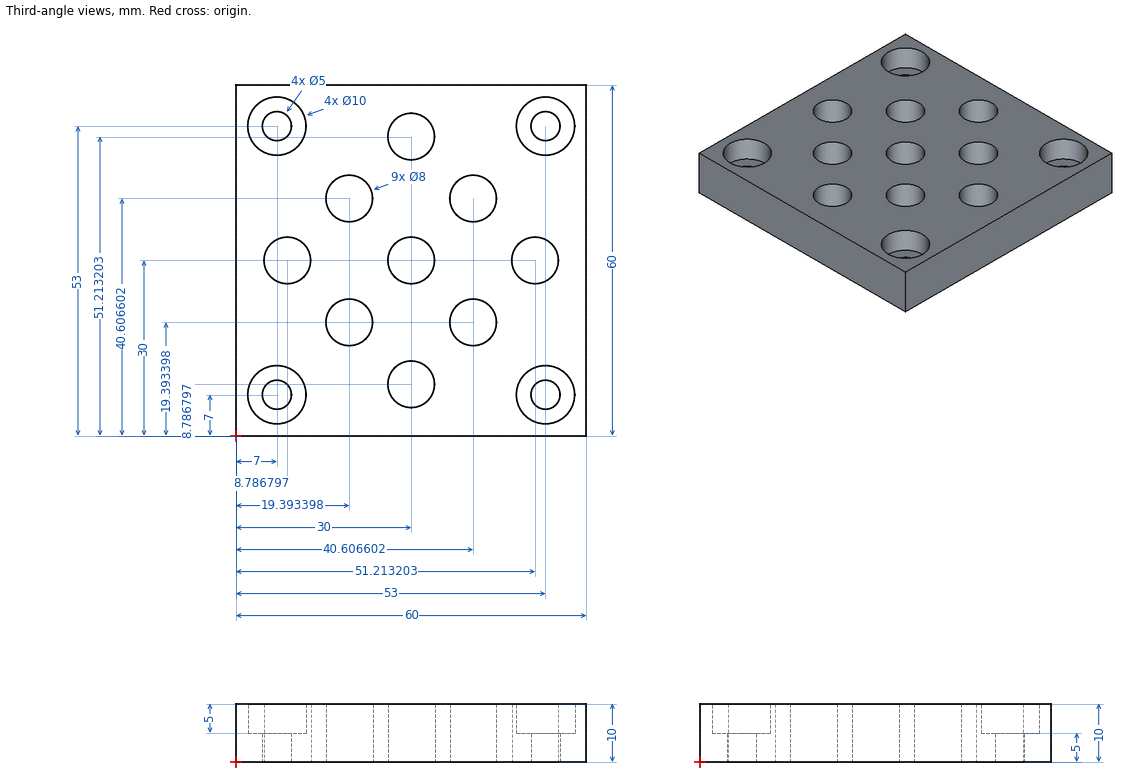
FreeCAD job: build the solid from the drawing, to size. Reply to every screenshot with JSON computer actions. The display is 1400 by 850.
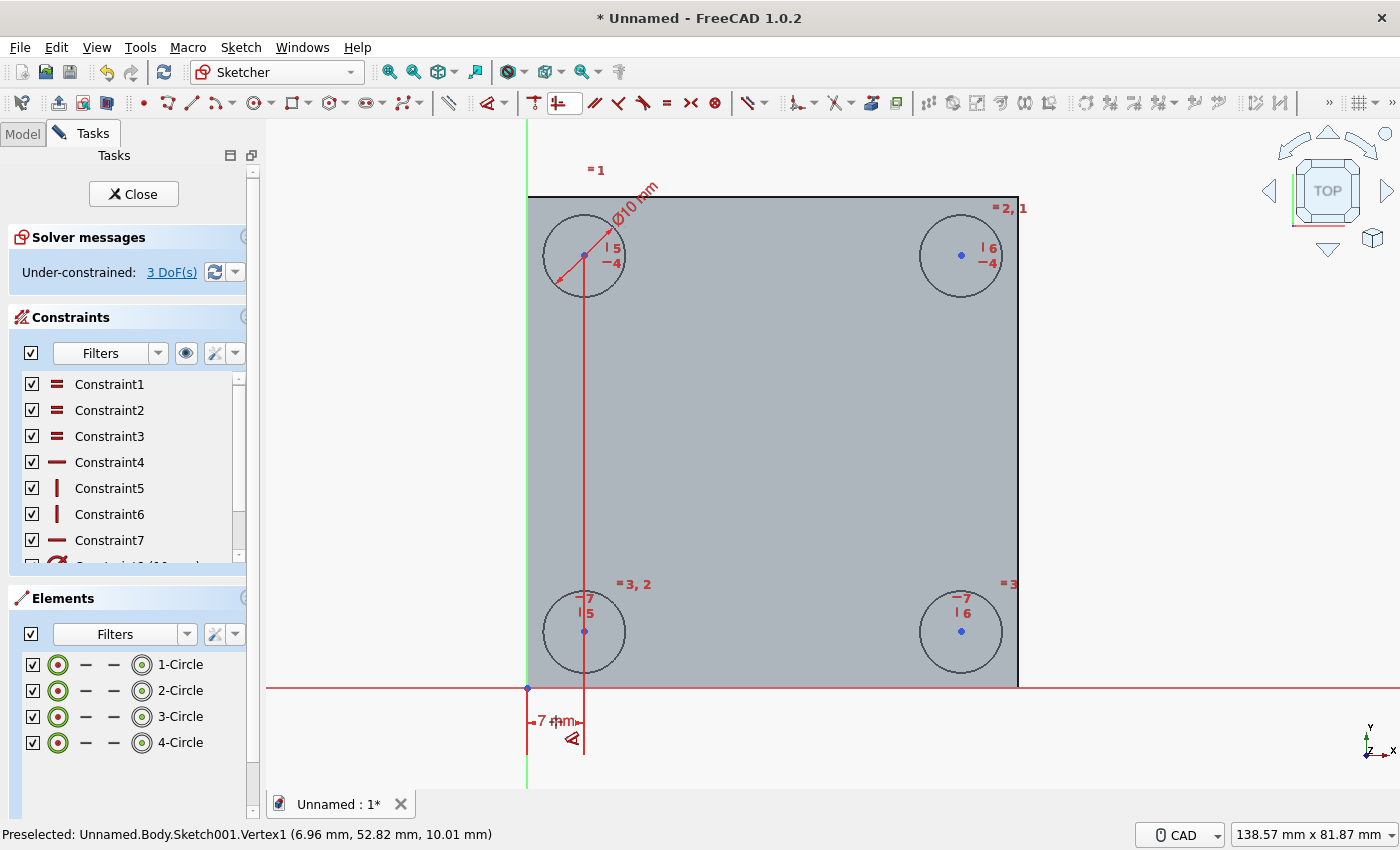
{"action": "left_click", "coordinate": [584, 632]}
{"action": "left_click", "coordinate": [493, 660]}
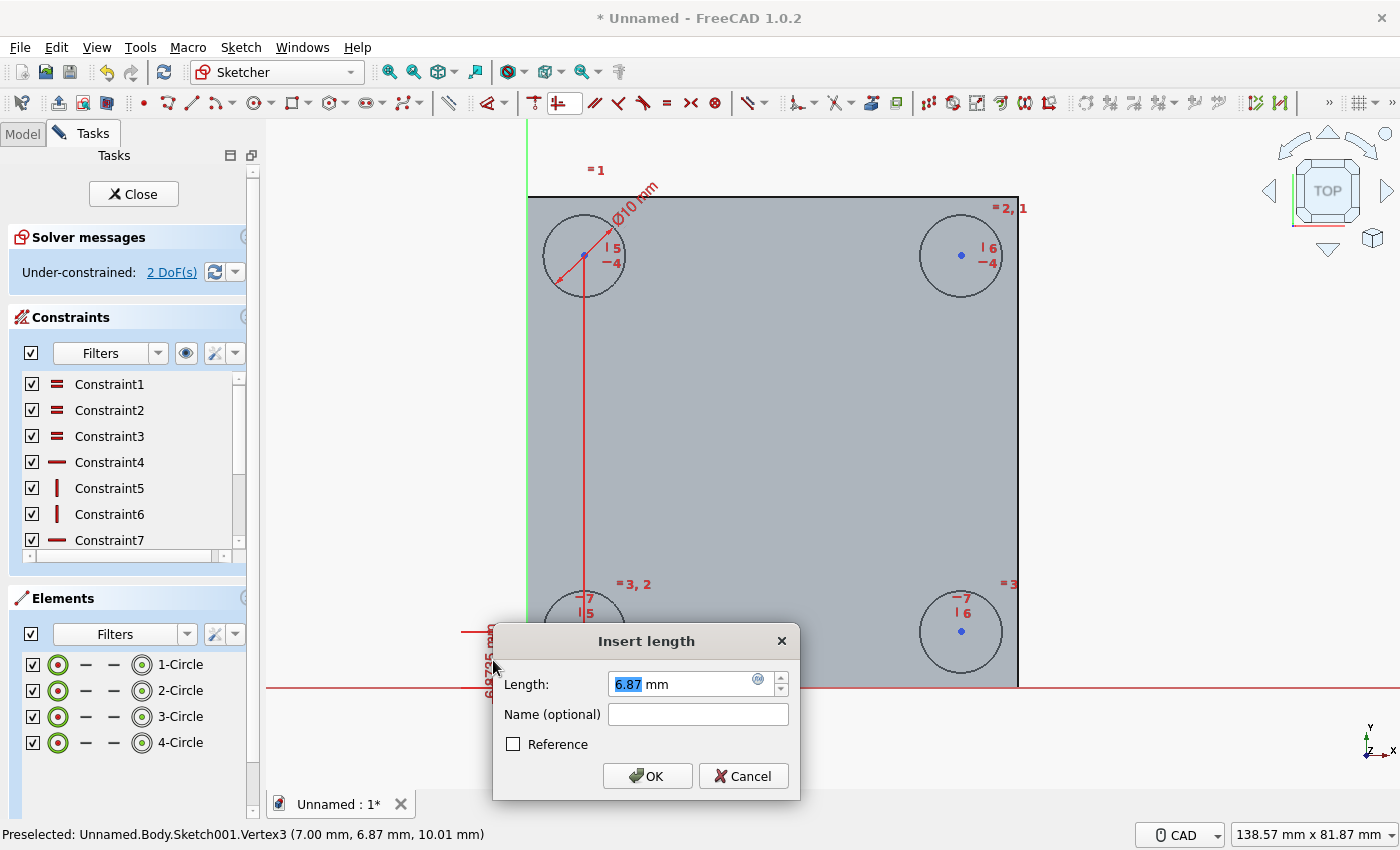
{"action": "type", "text": "7"}
{"action": "key", "text": "Return"}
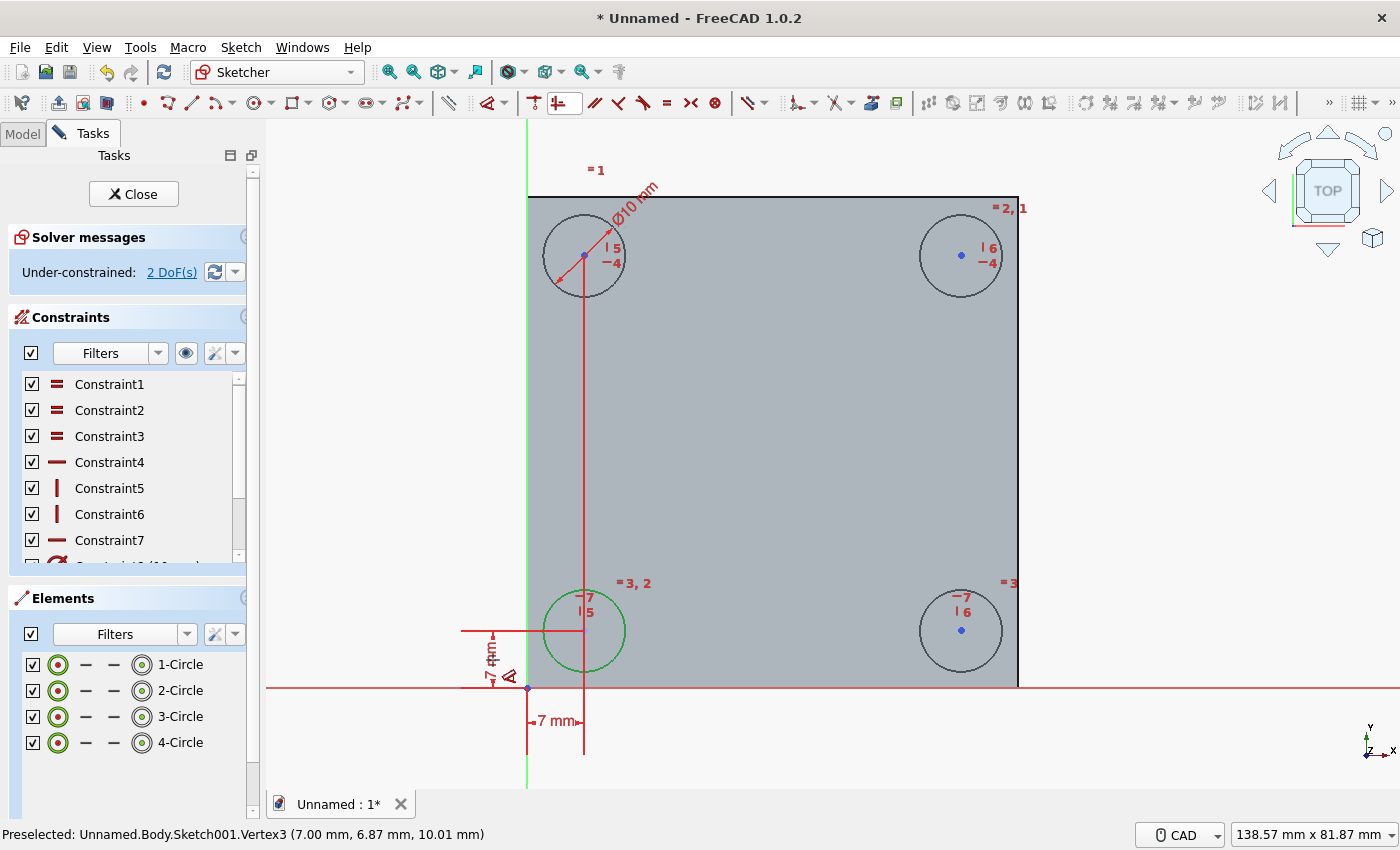
{"action": "left_click", "coordinate": [584, 256]}
{"action": "left_click", "coordinate": [493, 472]}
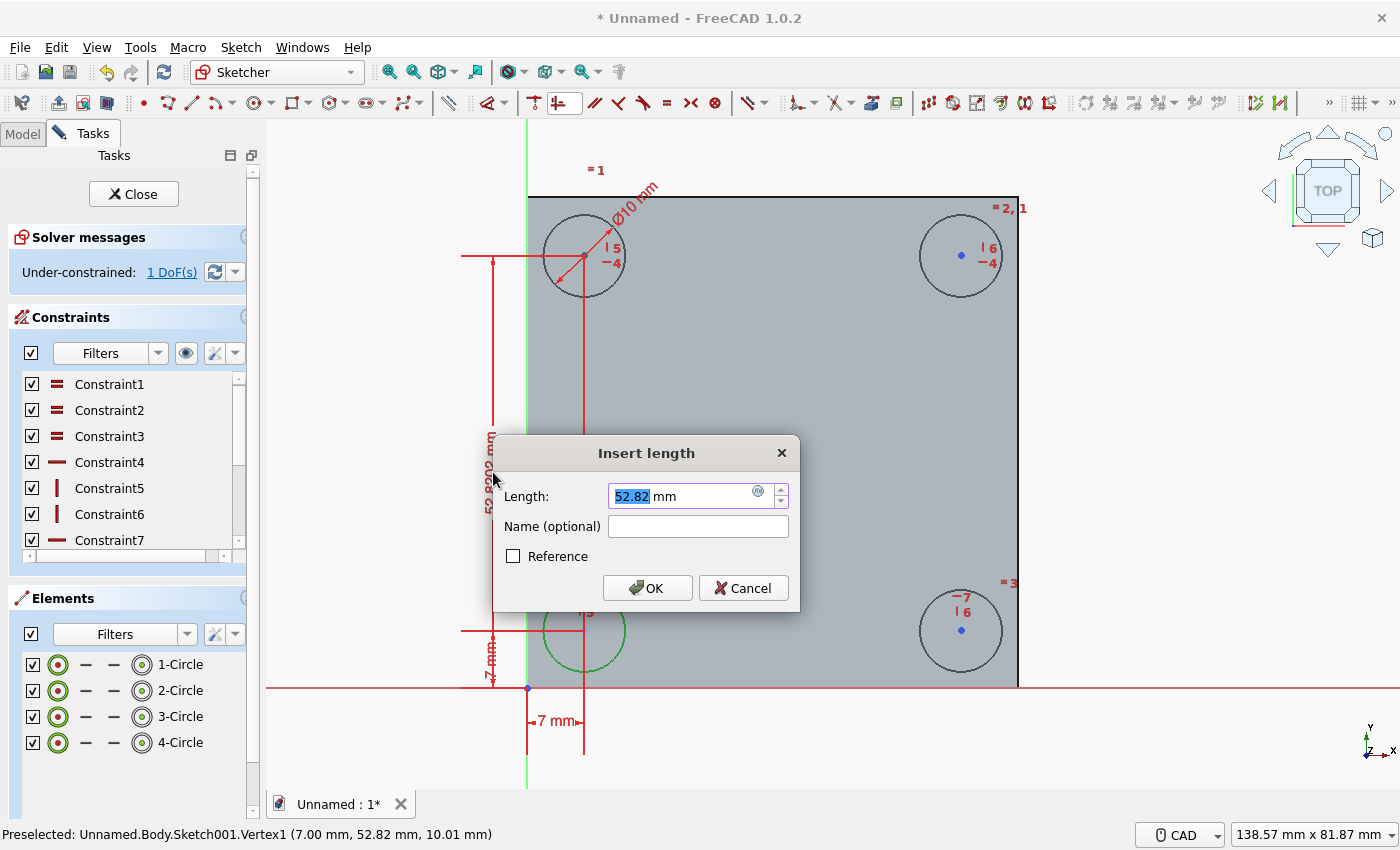
{"action": "type", "text": "53"}
{"action": "key", "text": "Return"}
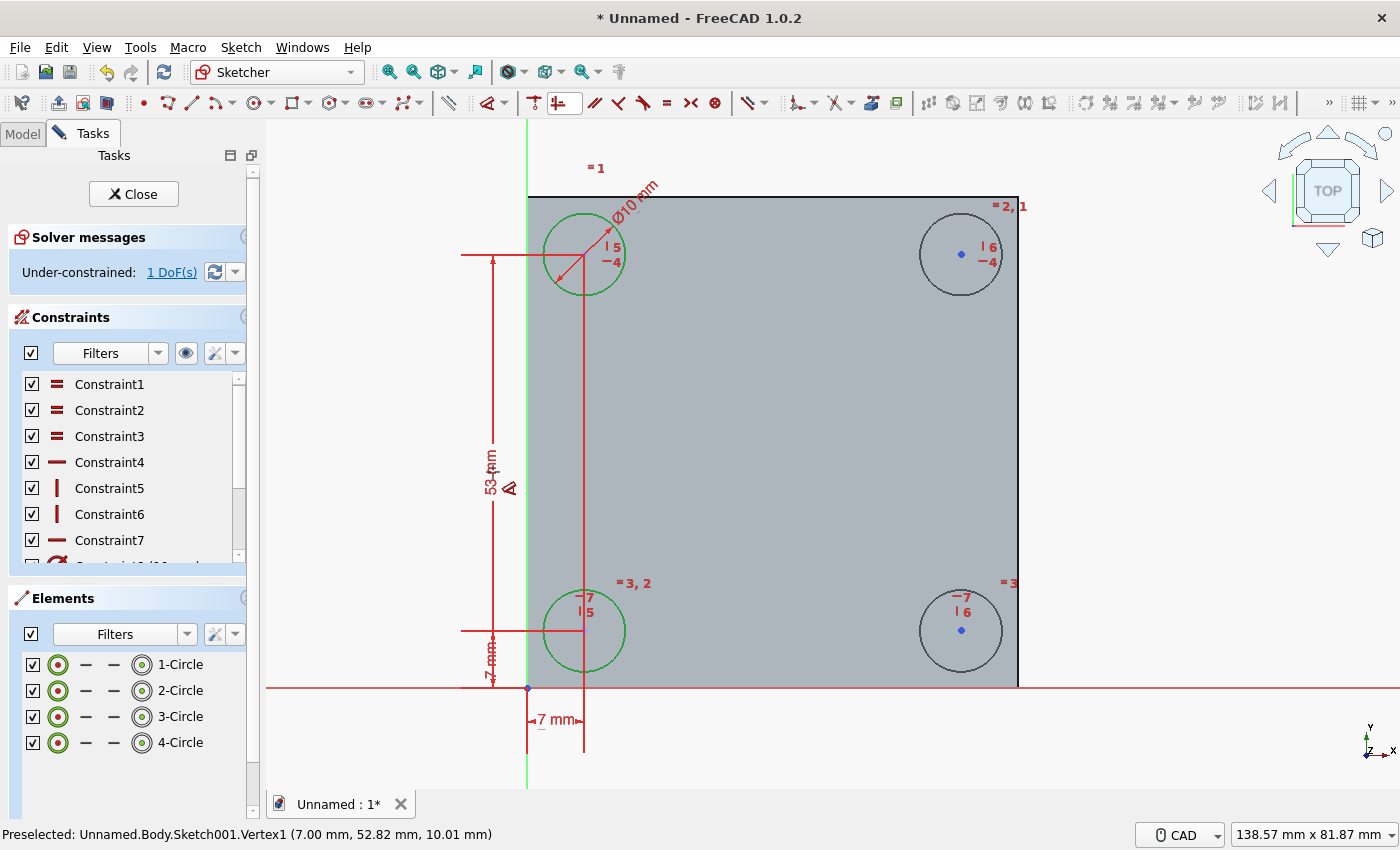
{"action": "left_click", "coordinate": [961, 255]}
{"action": "left_click", "coordinate": [744, 722]}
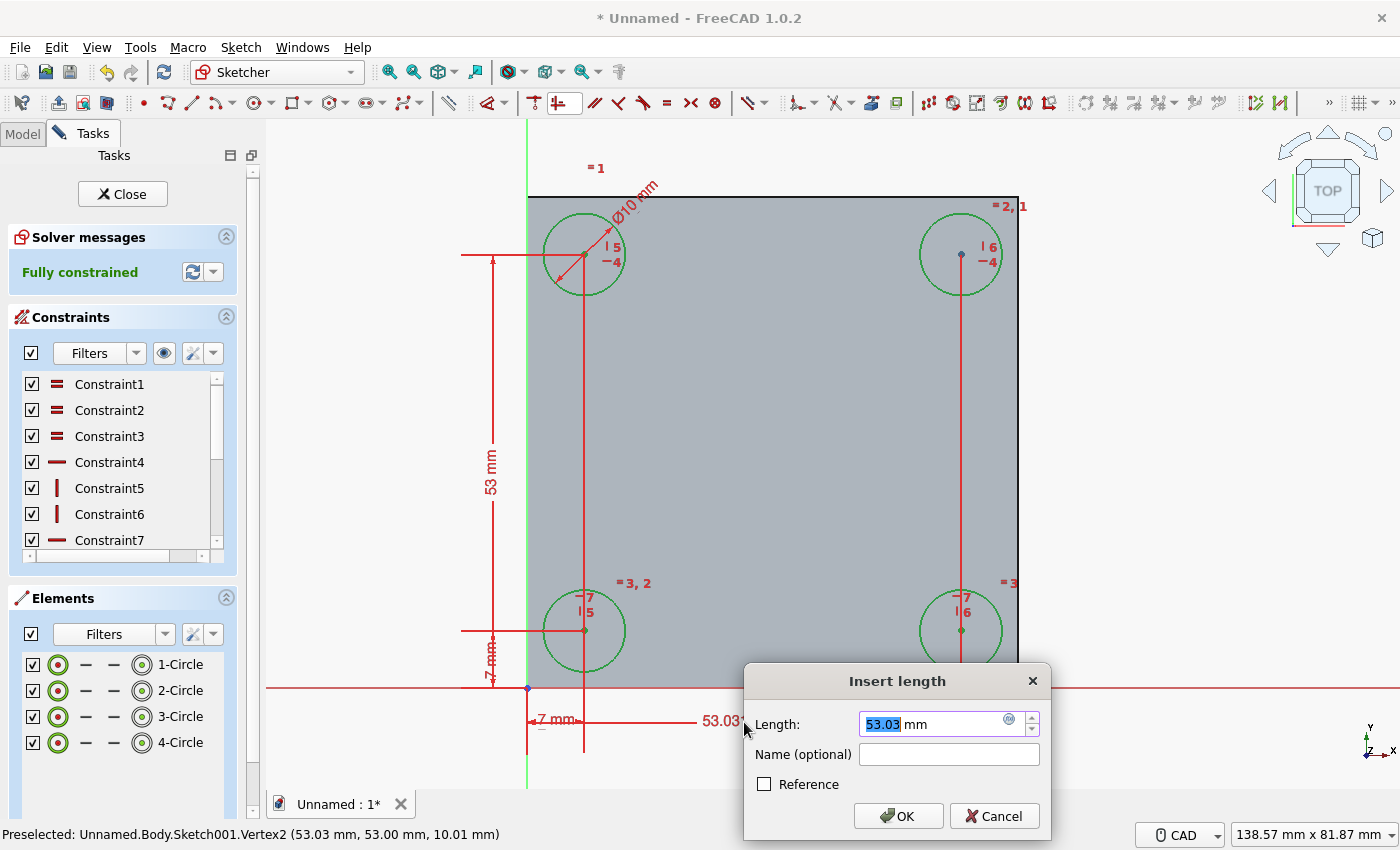
{"action": "type", "text": "53"}
{"action": "key", "text": "Return"}
{"action": "key", "text": "Escape"}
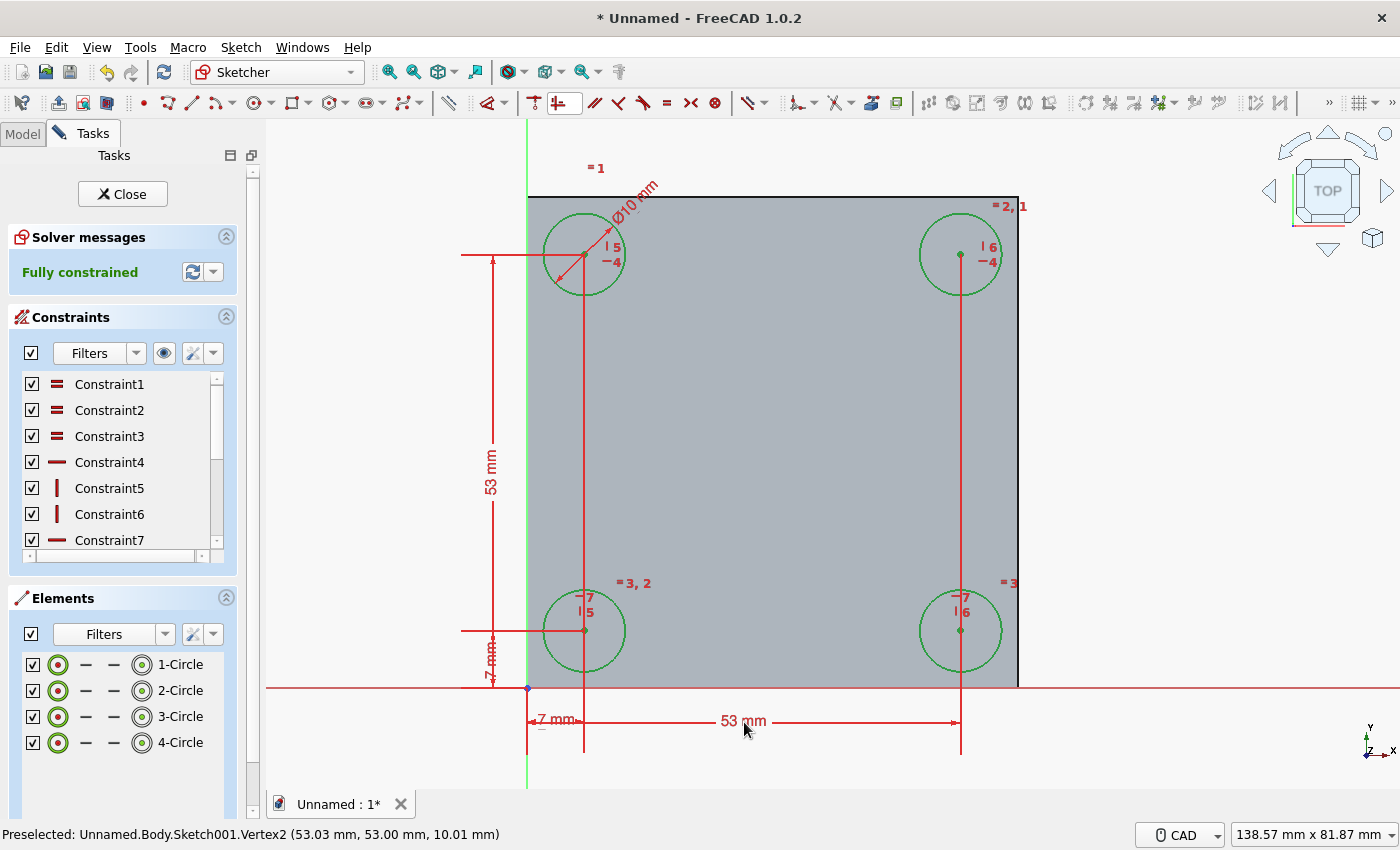
{"action": "left_click", "coordinate": [123, 194]}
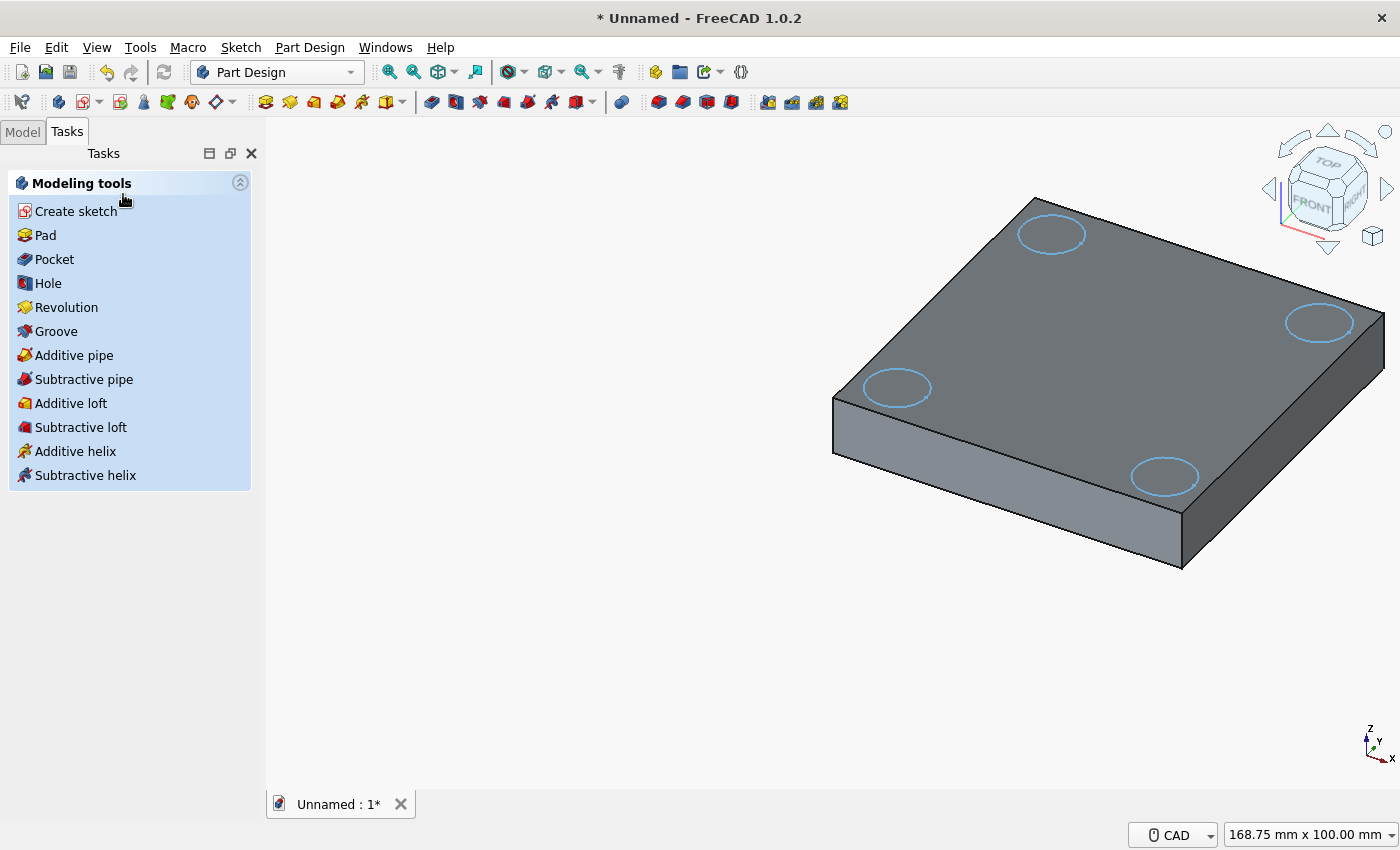
{"action": "left_click", "coordinate": [432, 102]}